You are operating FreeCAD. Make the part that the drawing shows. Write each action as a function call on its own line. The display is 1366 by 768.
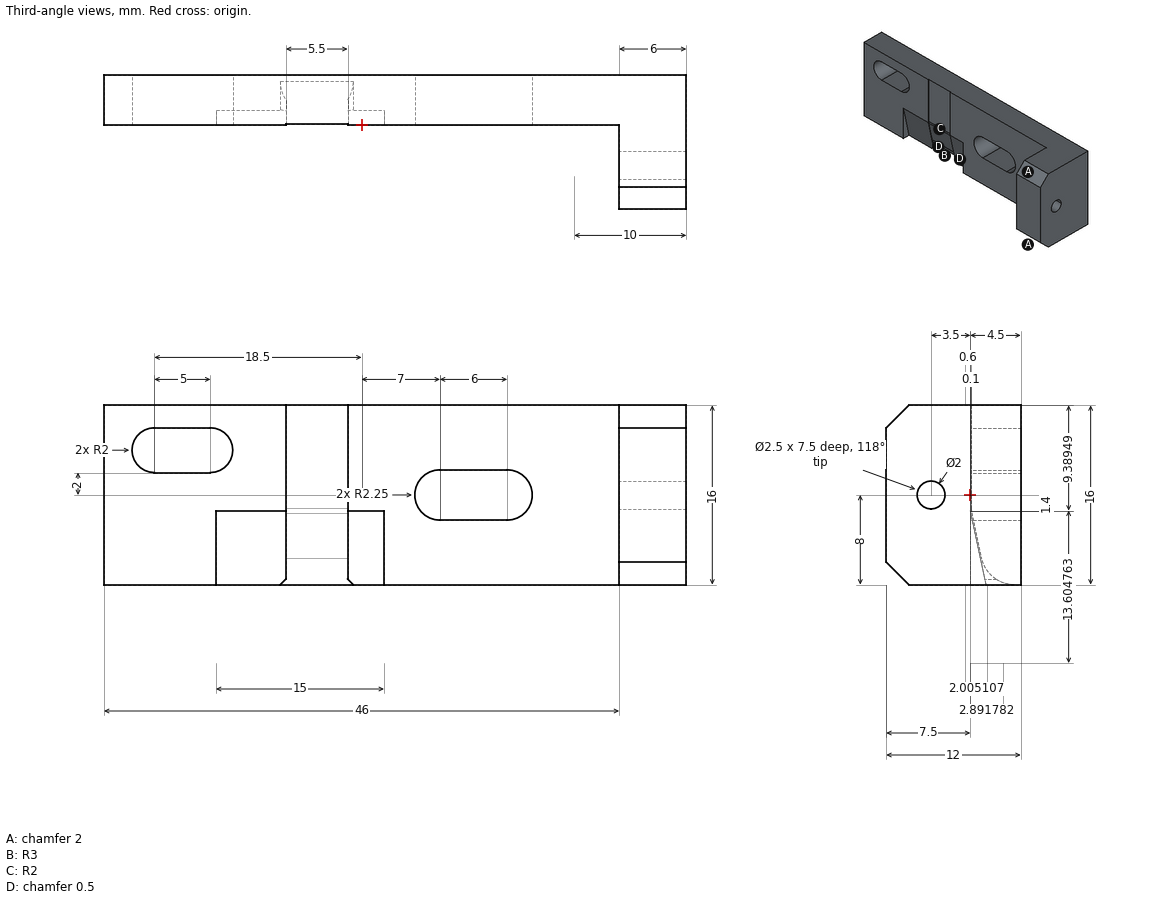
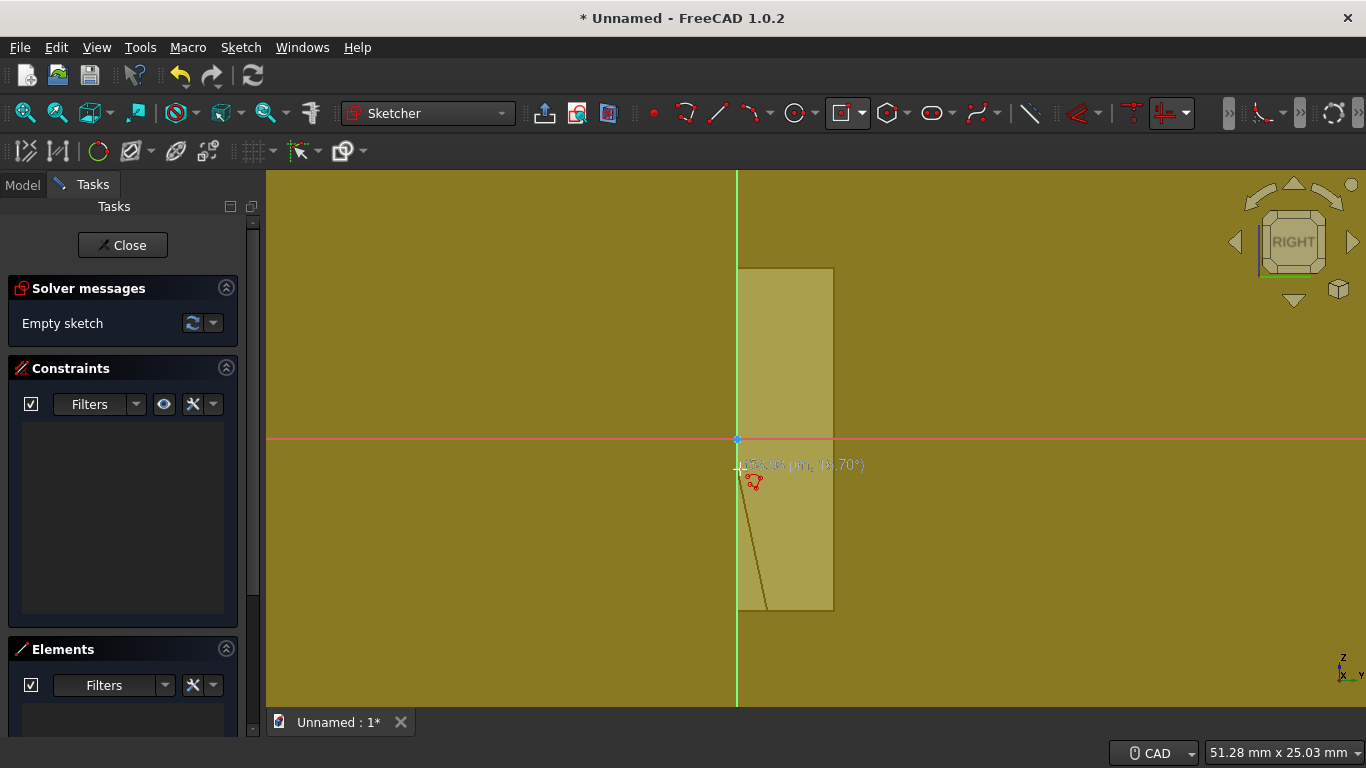
click(769, 611)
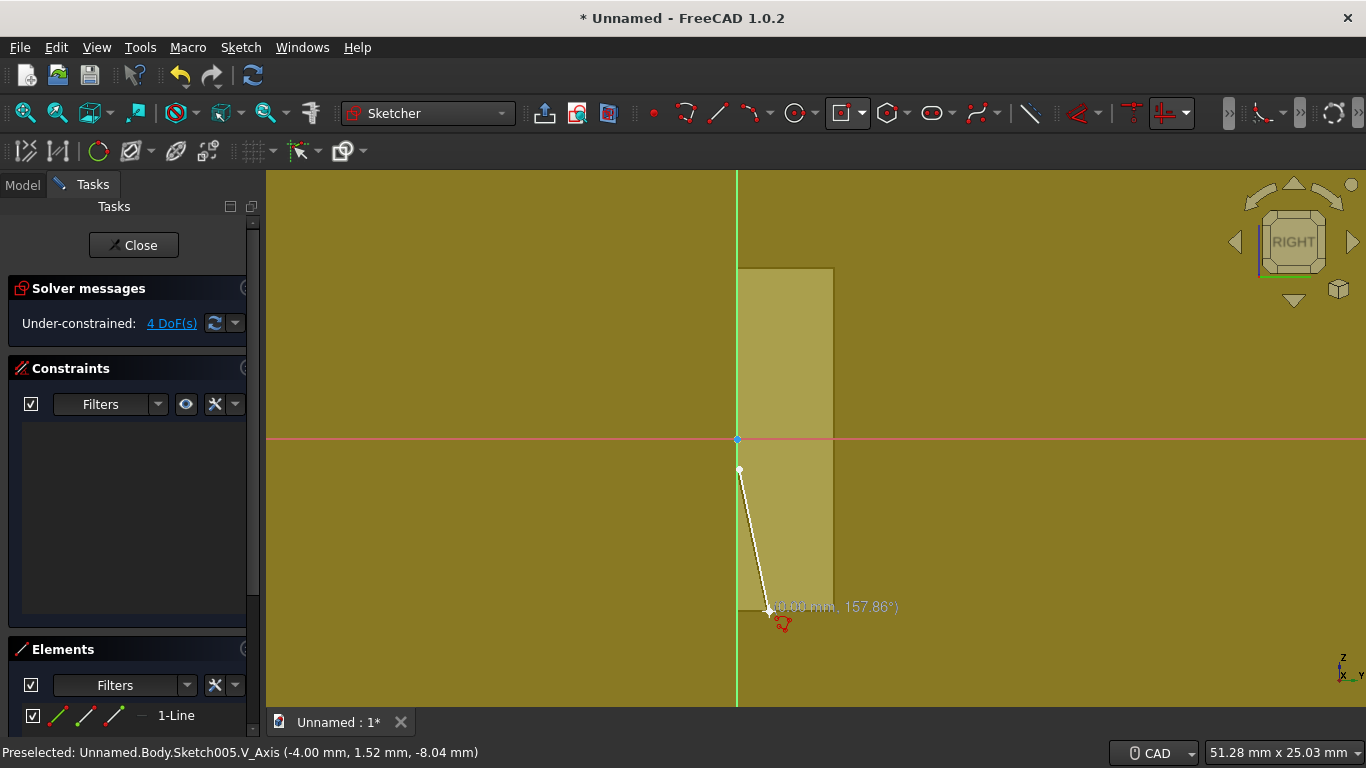
scroll(726, 611, up, 2)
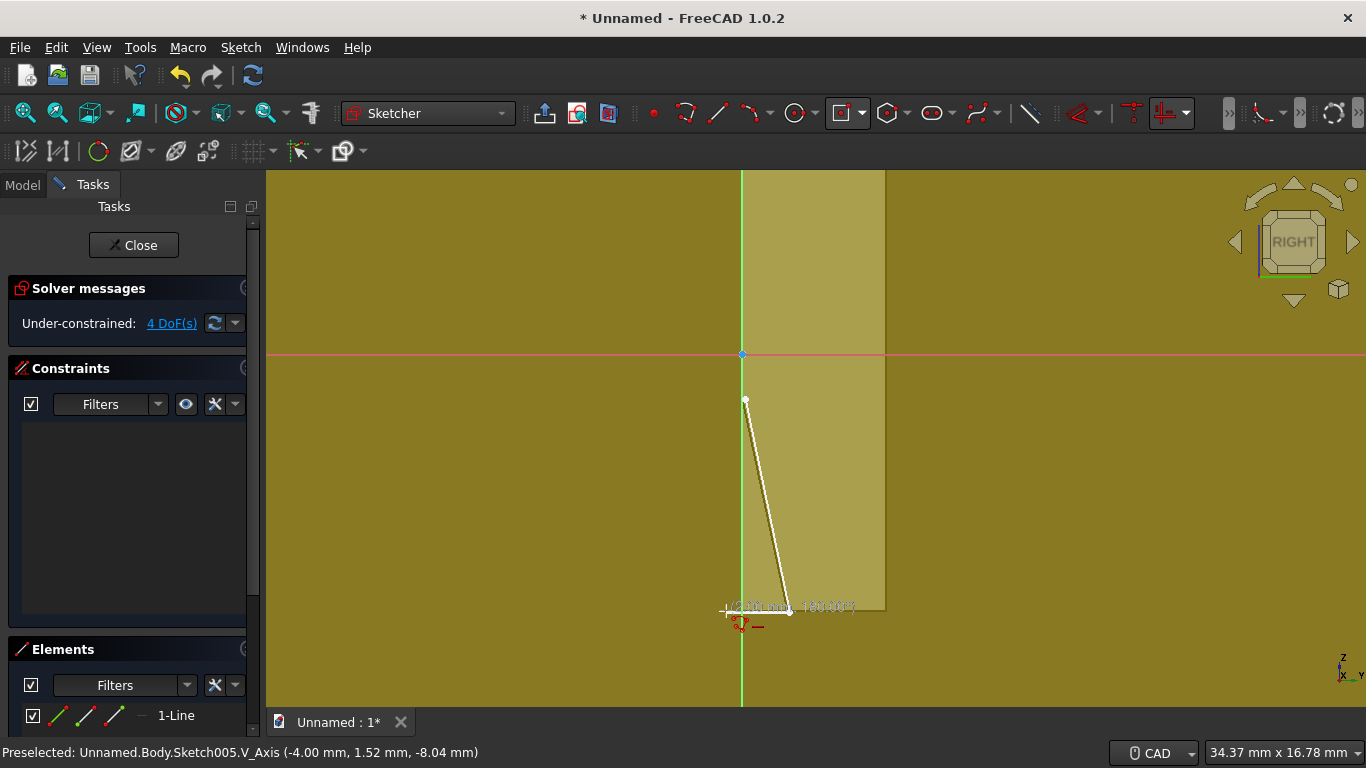
click(726, 611)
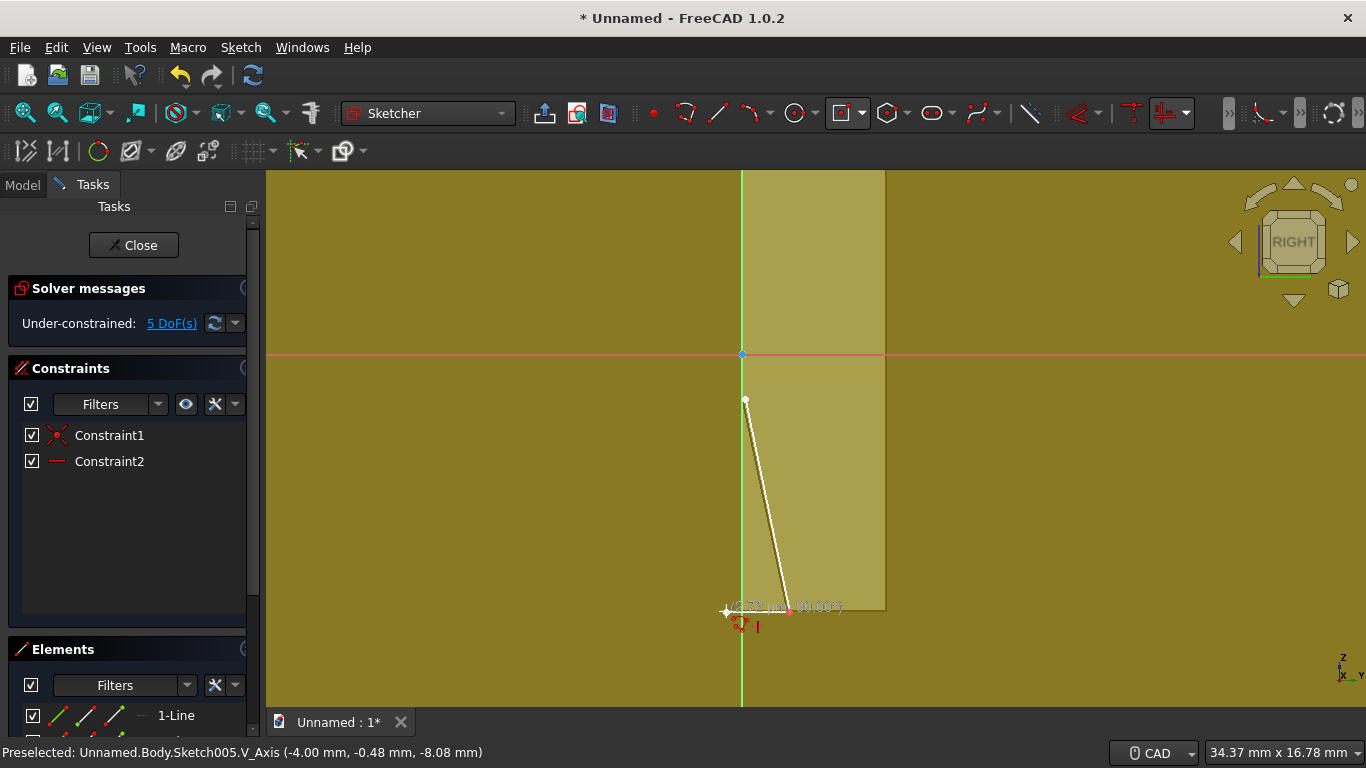
scroll(725, 609, down, 2)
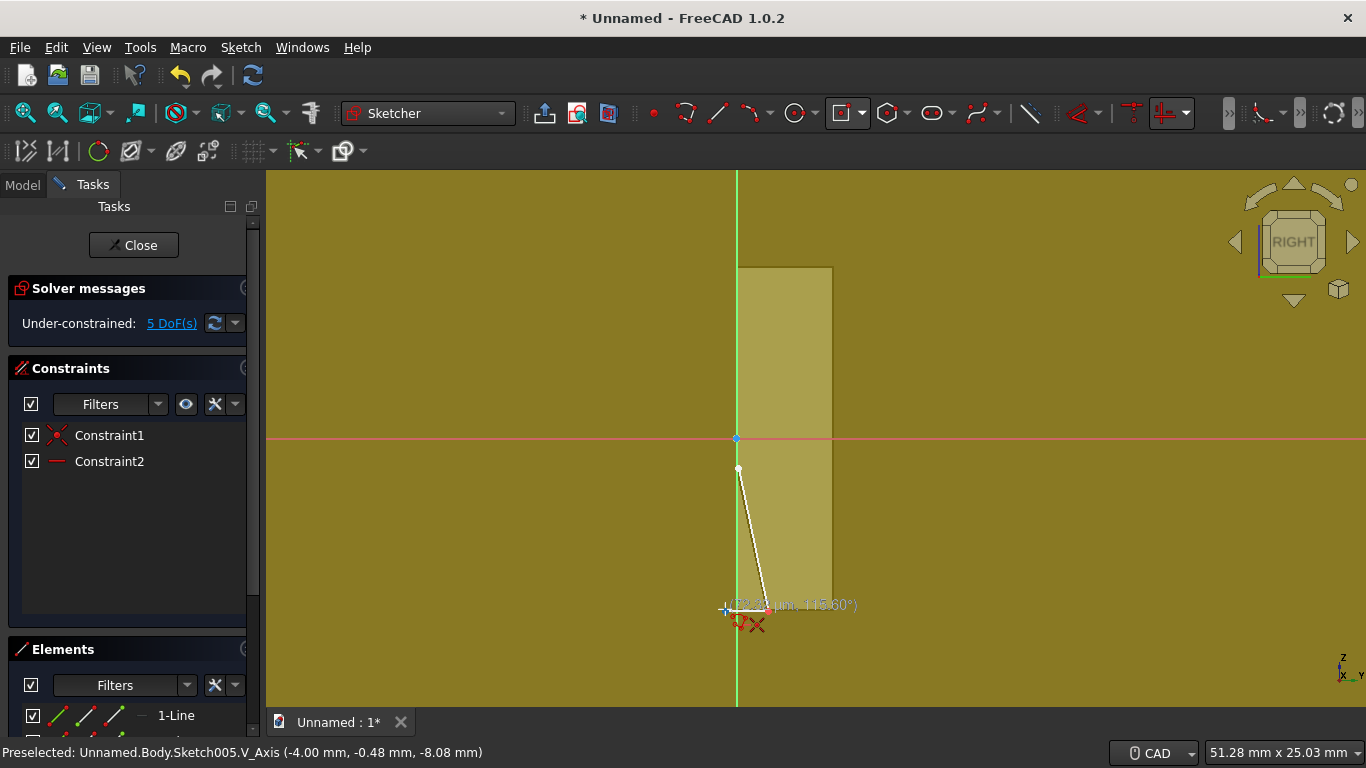
scroll(726, 267, up, 2)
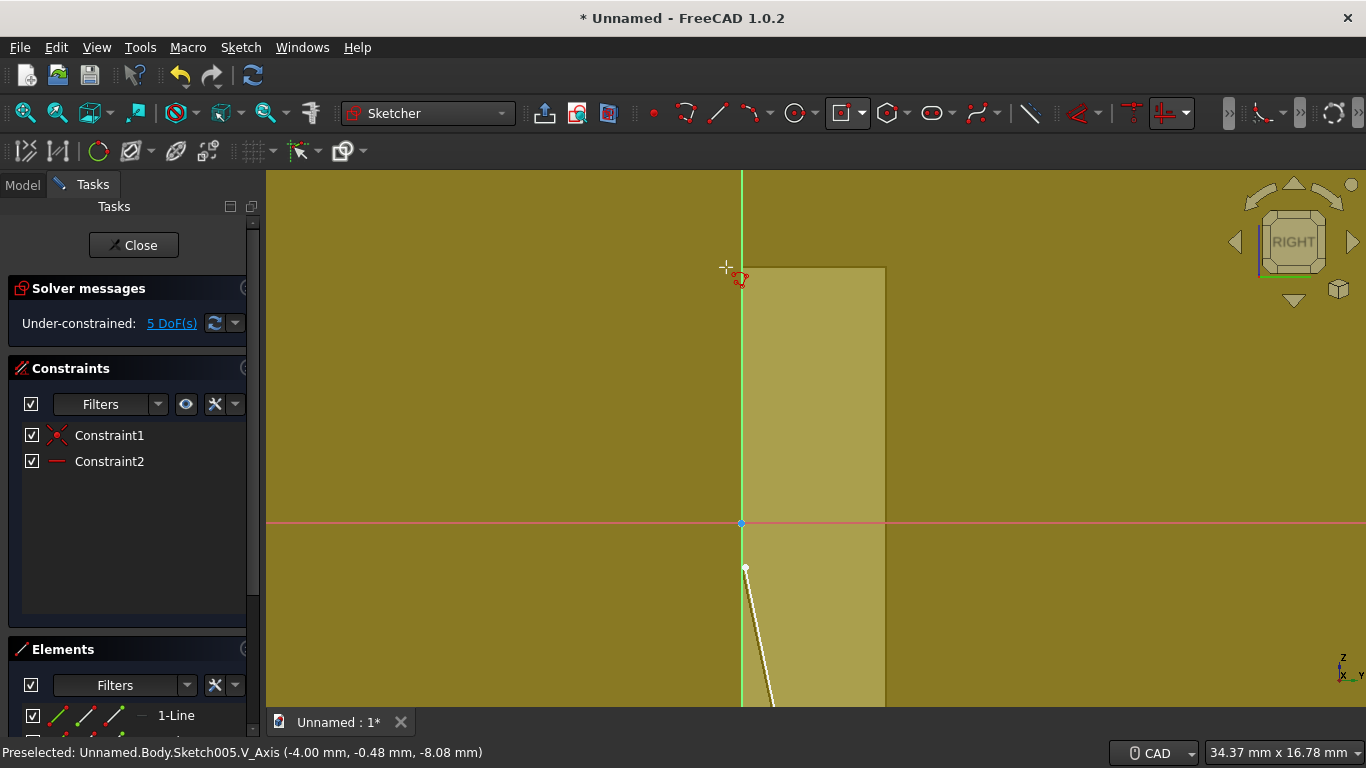
click(726, 267)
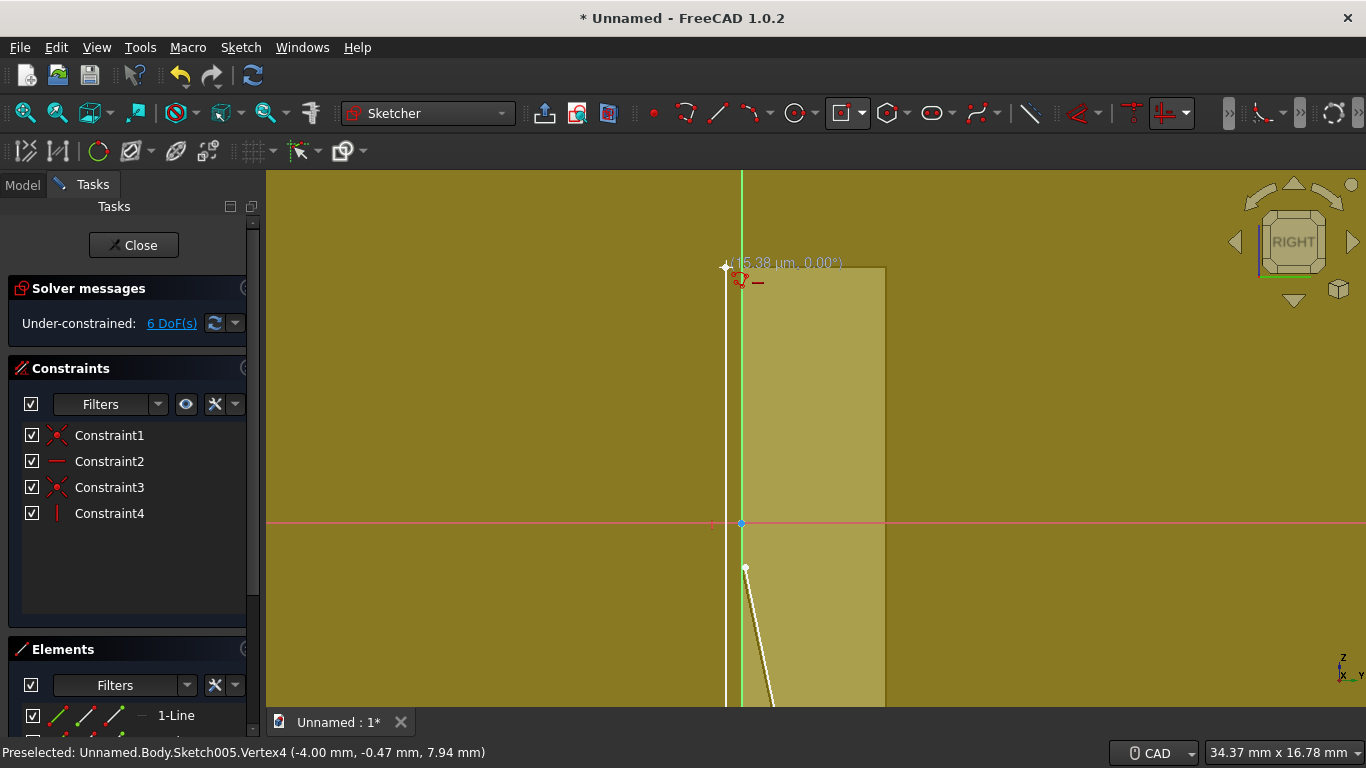
scroll(745, 267, up, 9)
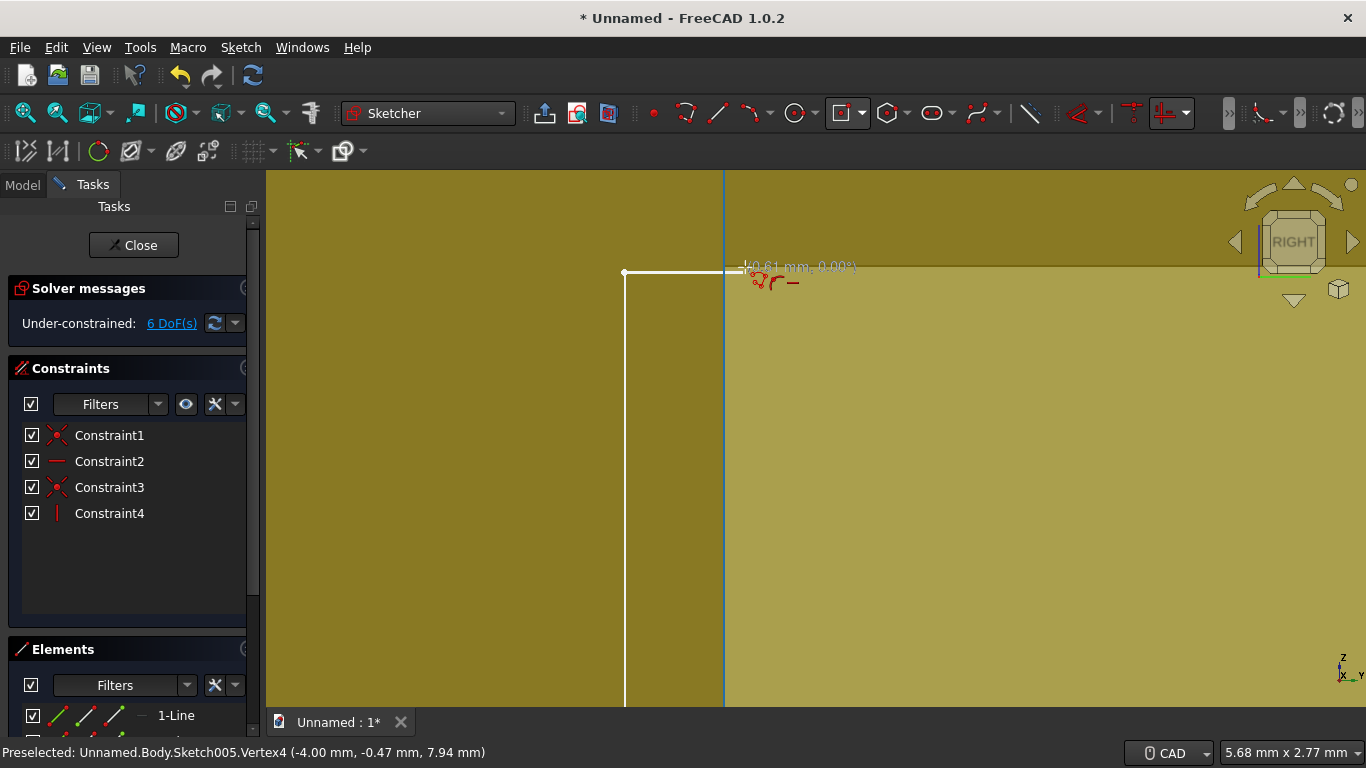
click(744, 266)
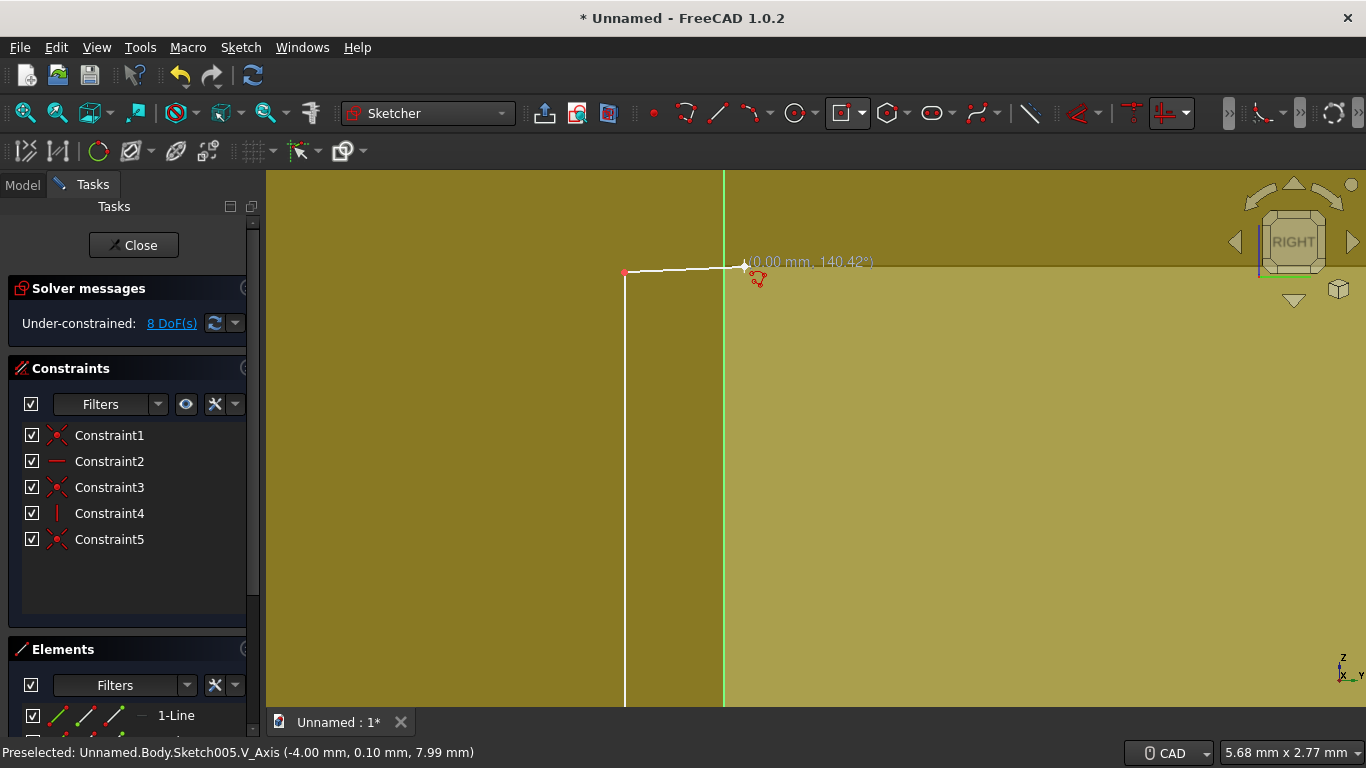
scroll(738, 267, down, 11)